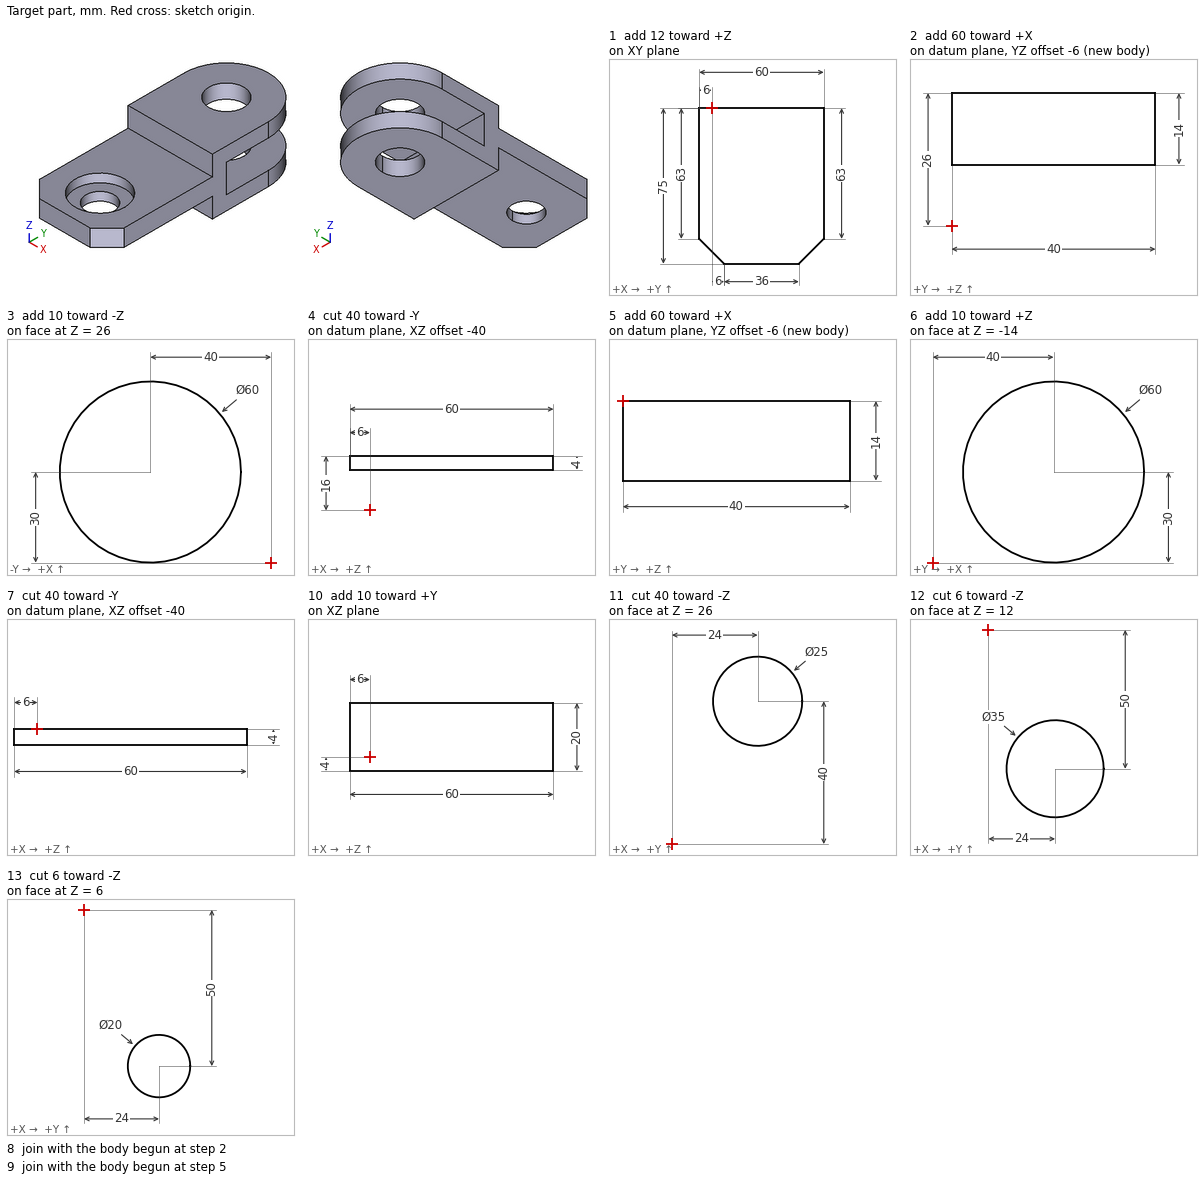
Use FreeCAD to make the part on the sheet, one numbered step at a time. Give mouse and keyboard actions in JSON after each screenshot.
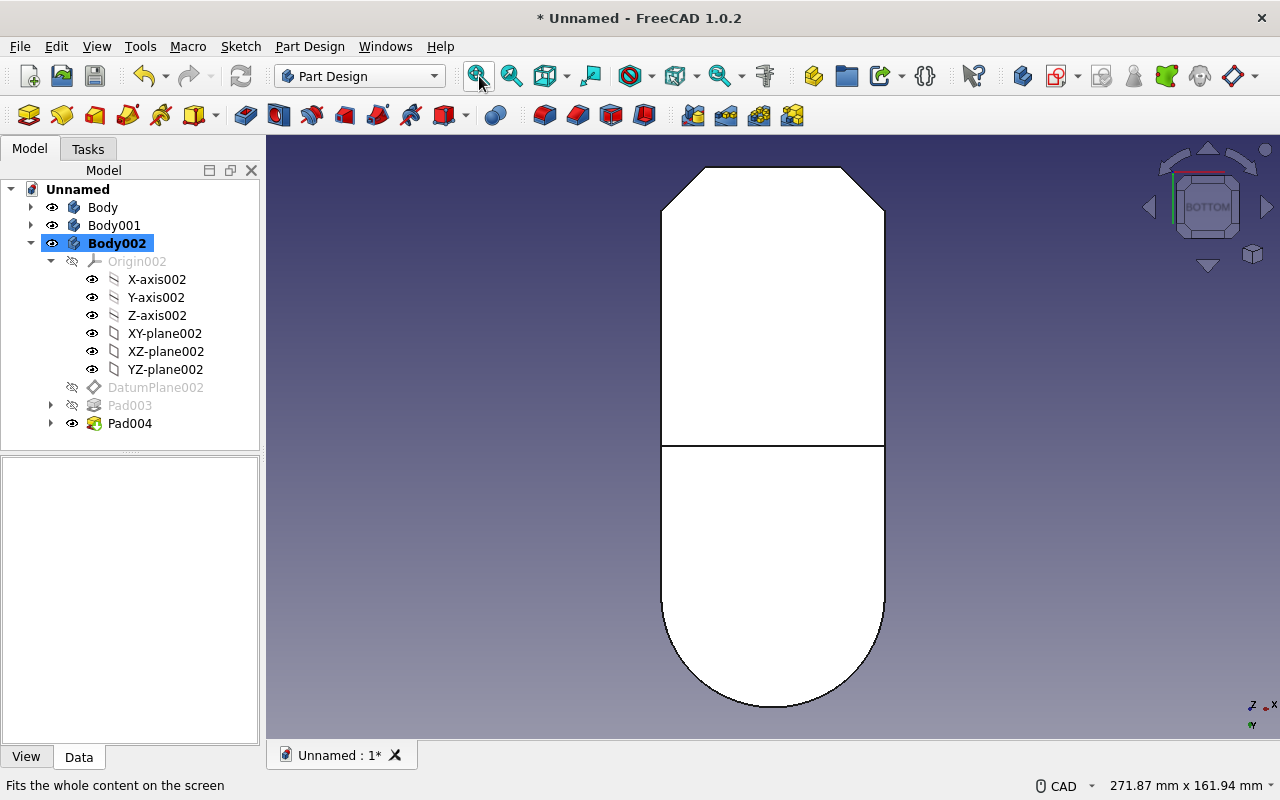
{"action": "left_click", "coordinate": [479, 76]}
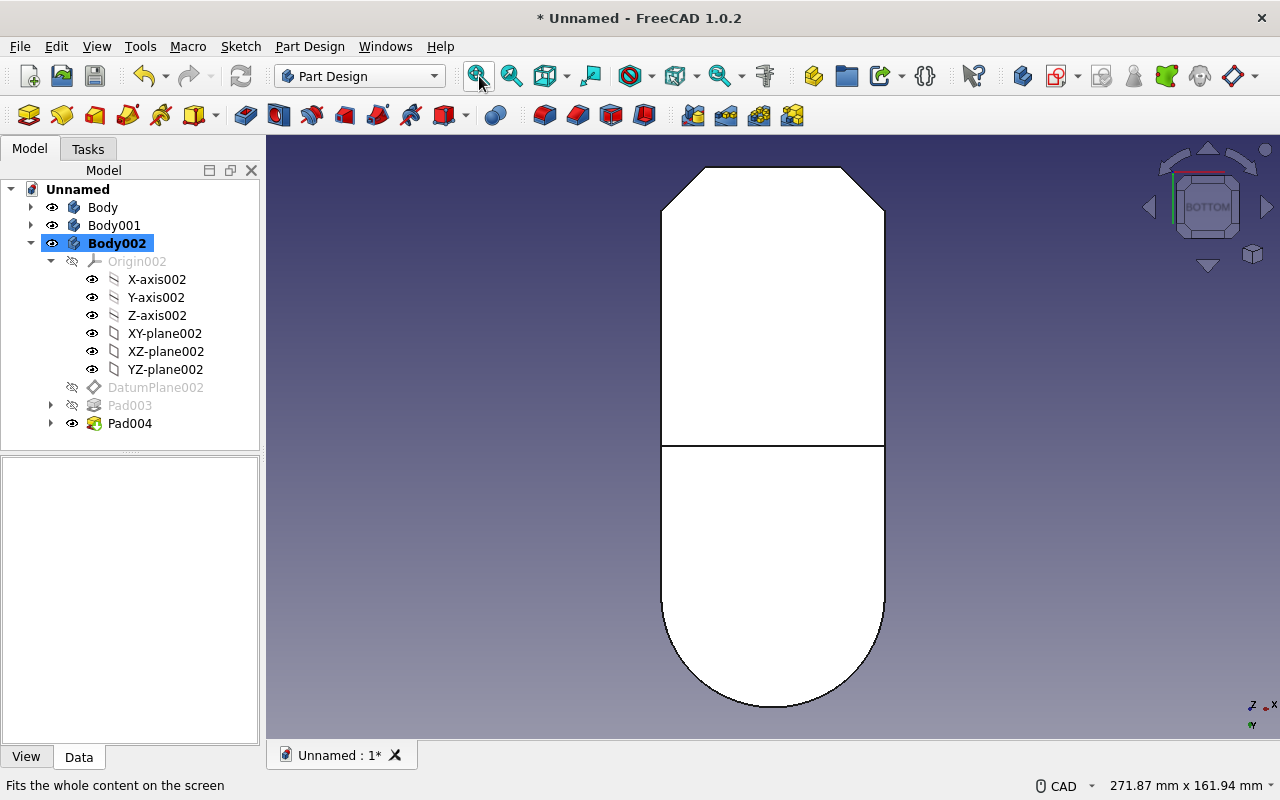
{"action": "key", "text": "3"}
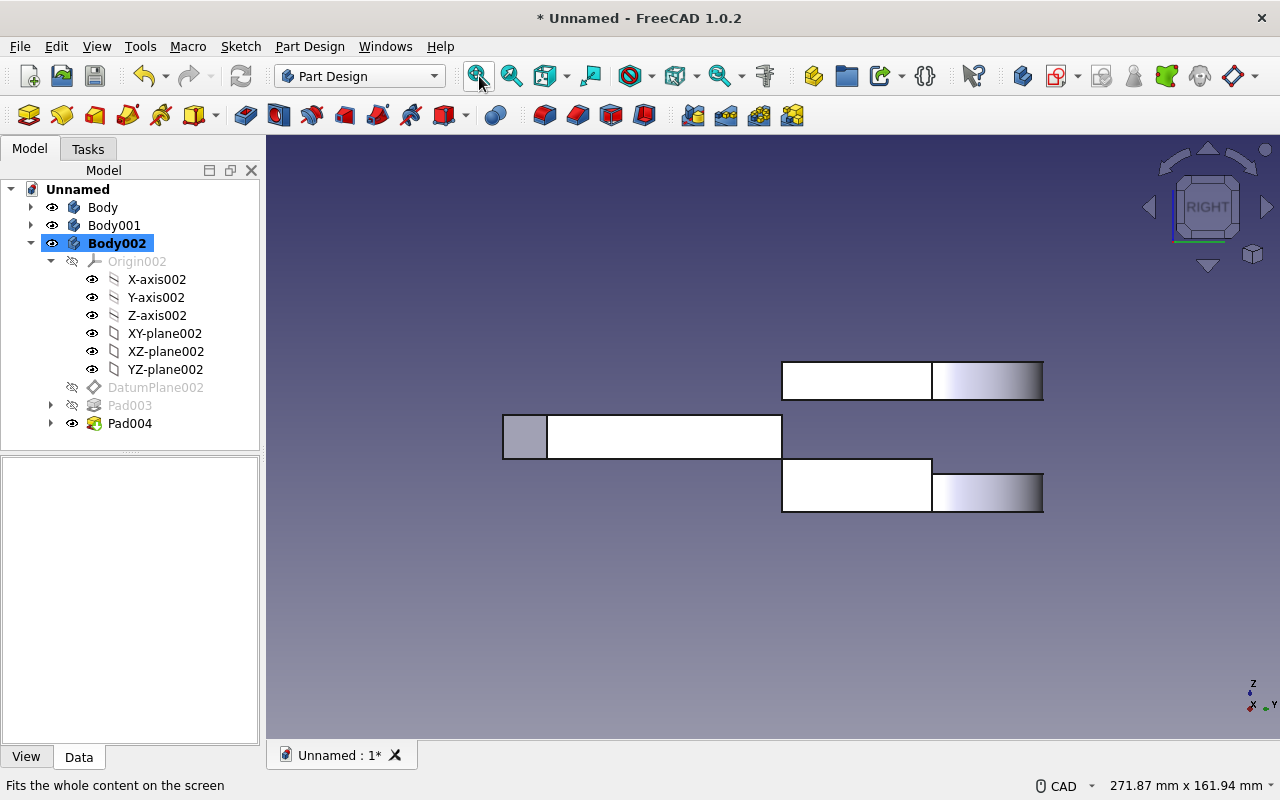
{"action": "left_click", "coordinate": [479, 76]}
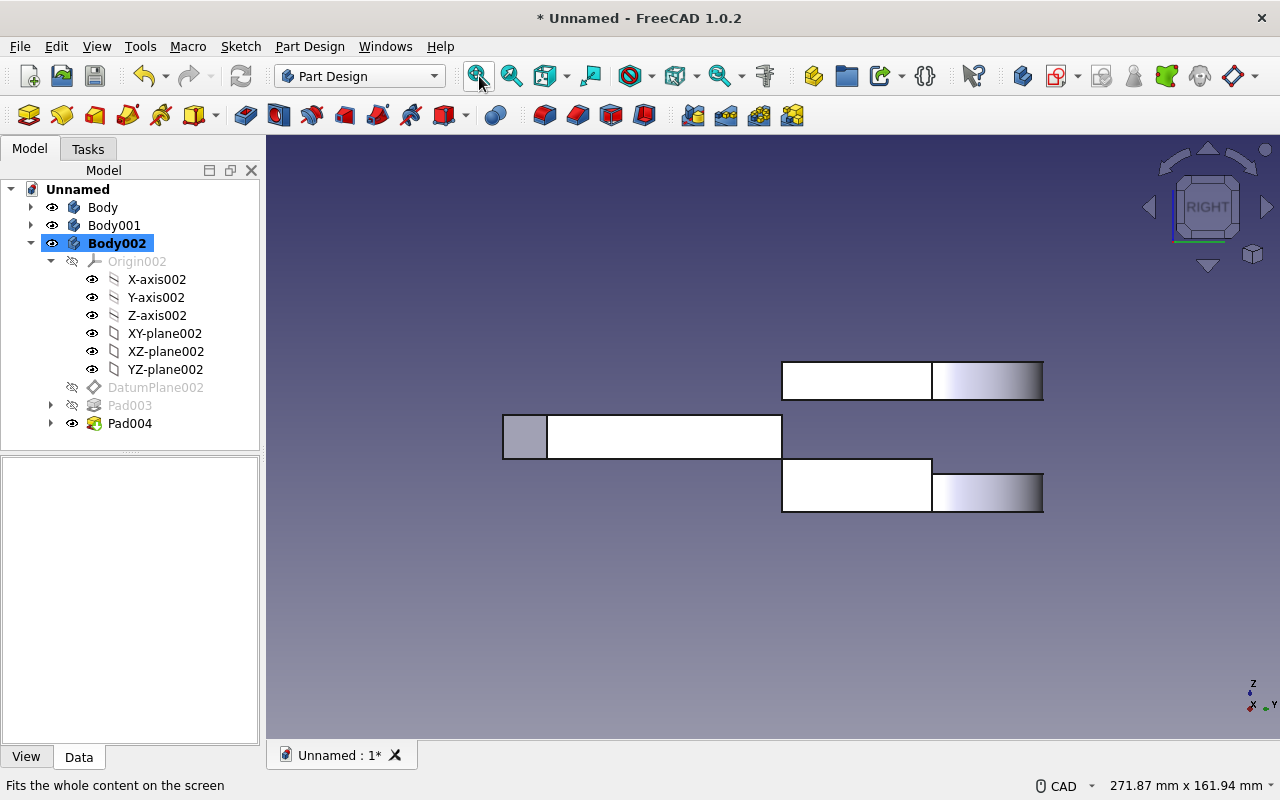
{"action": "left_click", "coordinate": [137, 351]}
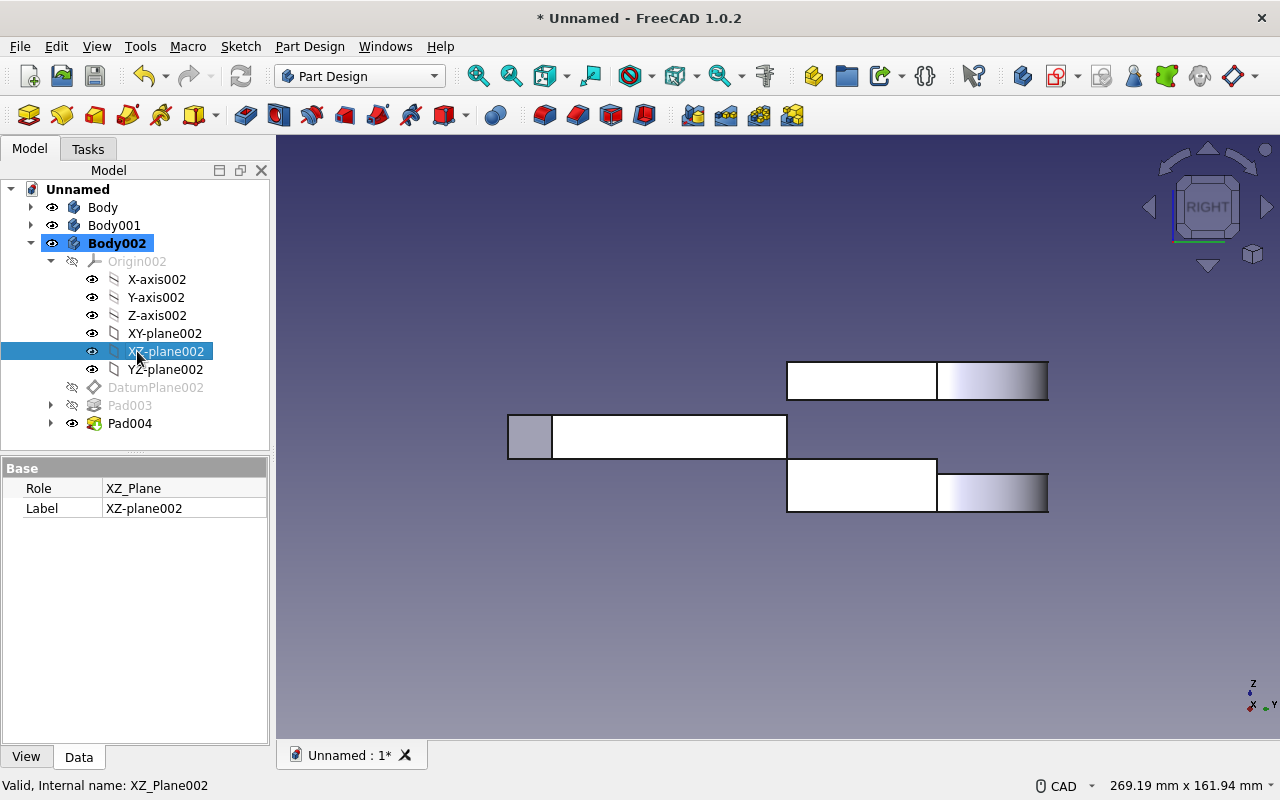
{"action": "left_click", "coordinate": [1232, 76]}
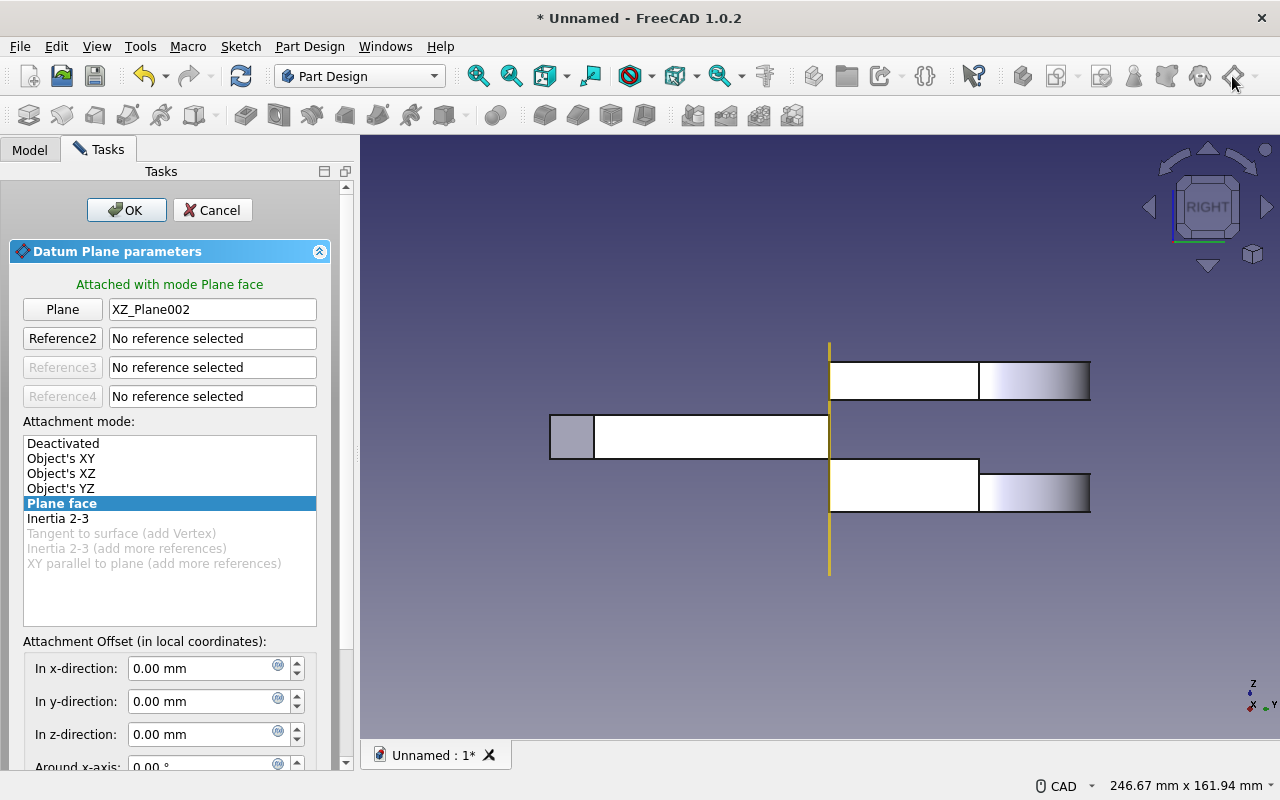
{"action": "triple_click", "coordinate": [210, 734]}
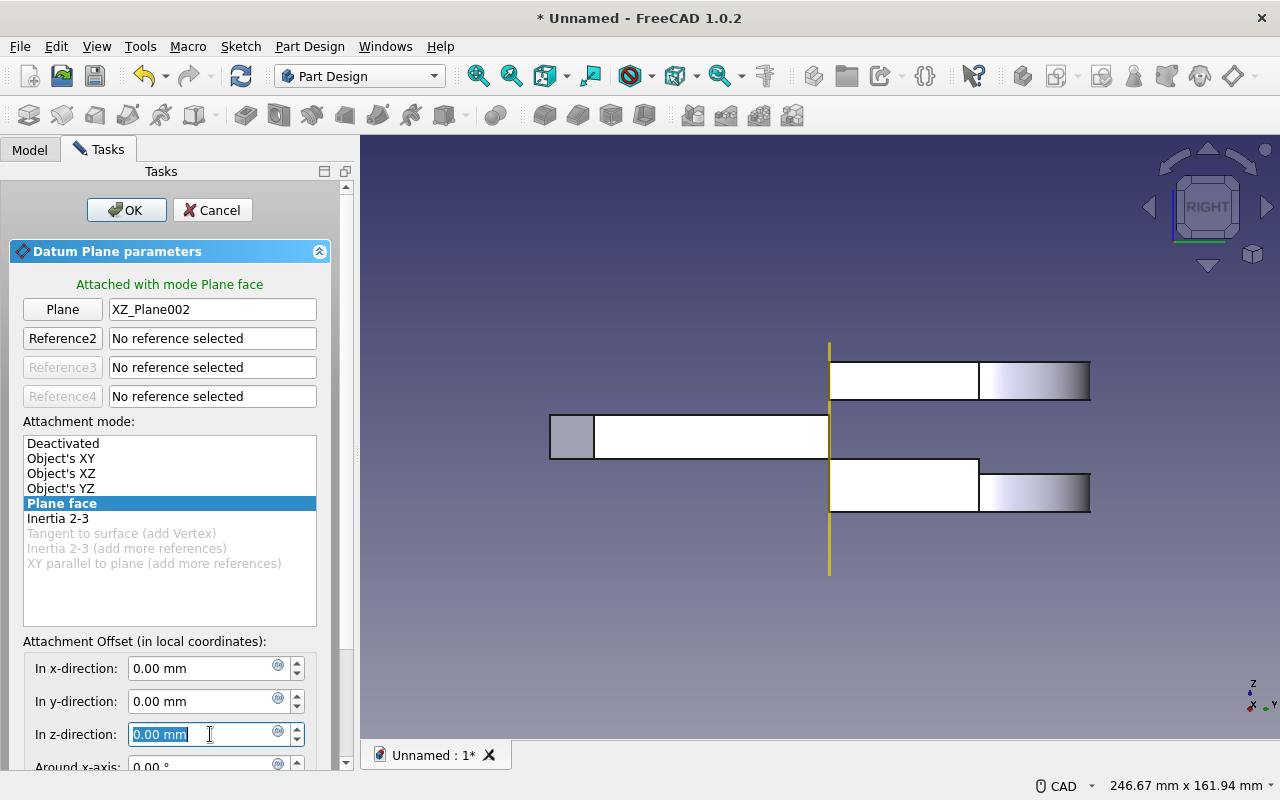
{"action": "type", "text": "-40"}
{"action": "key", "text": "Tab"}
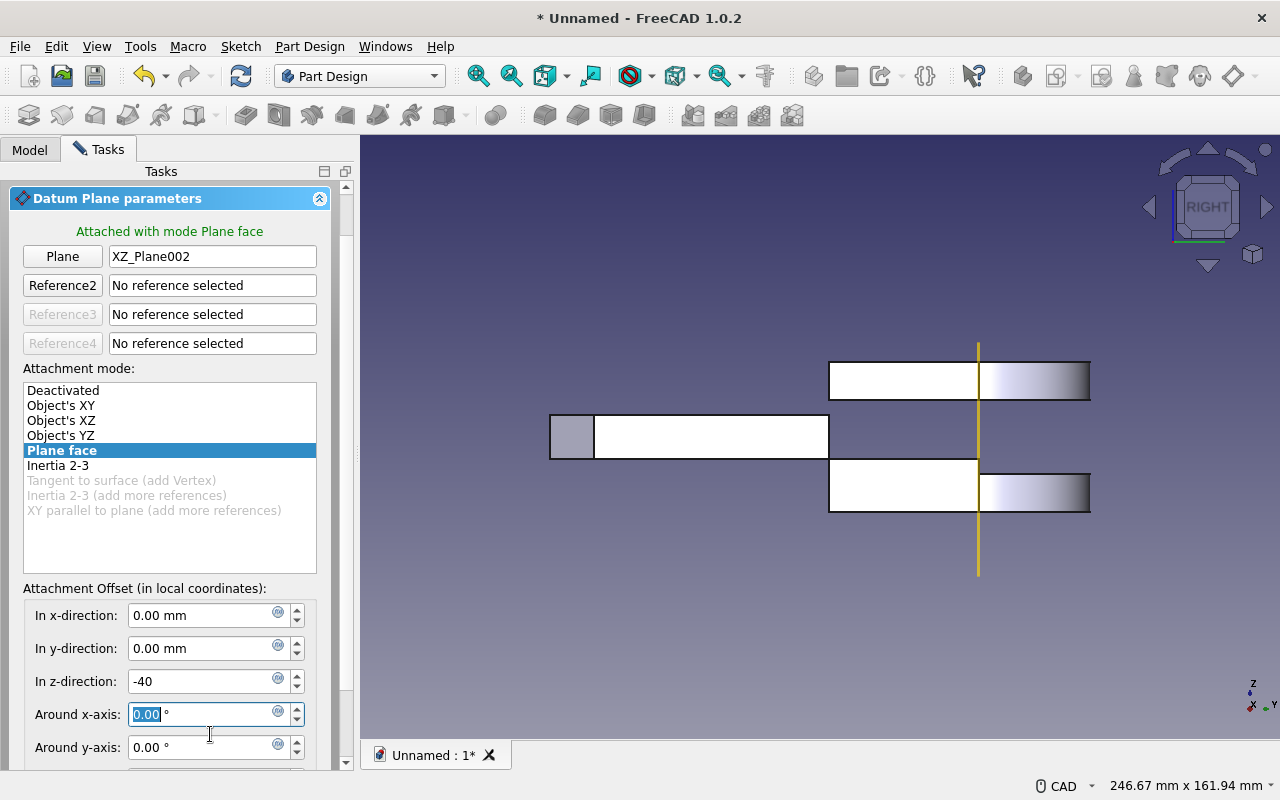
{"action": "scroll", "coordinate": [346, 476], "scroll_direction": "up", "scroll_amount": 2}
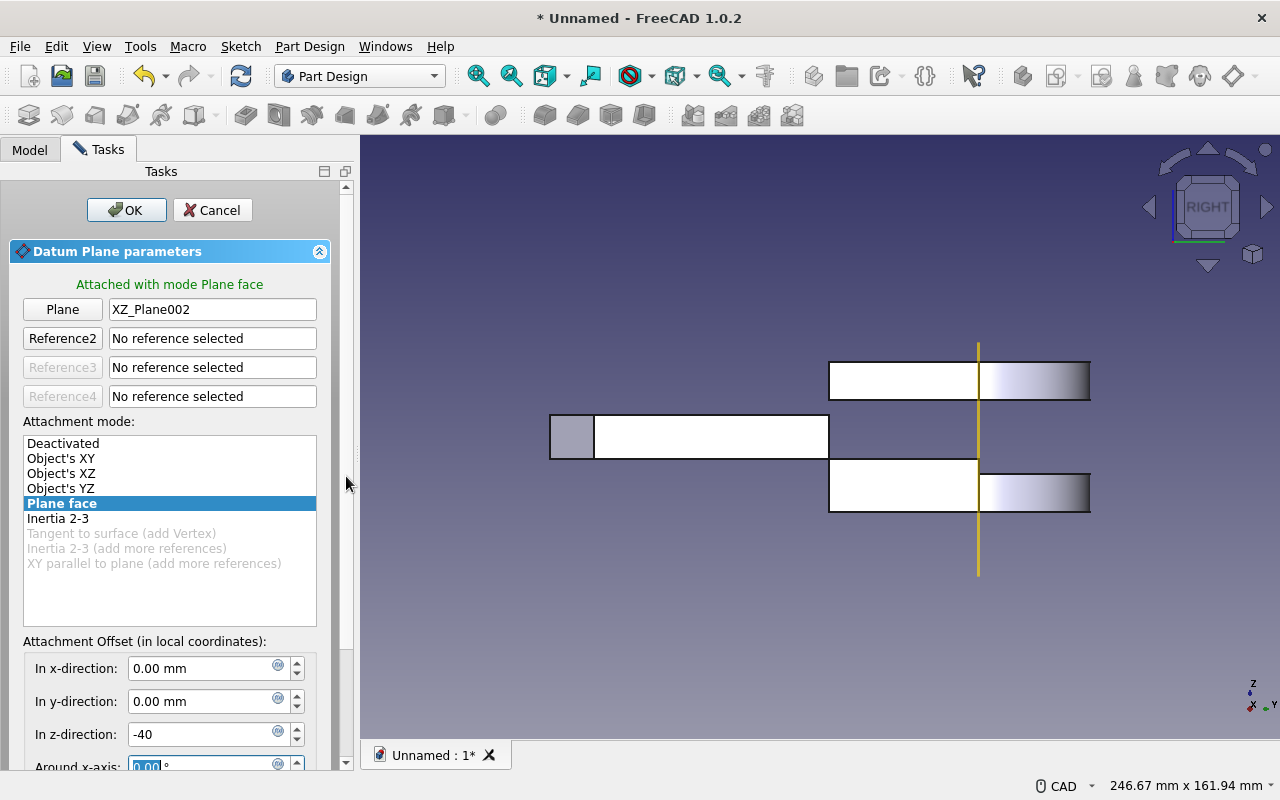
{"action": "left_click", "coordinate": [127, 210]}